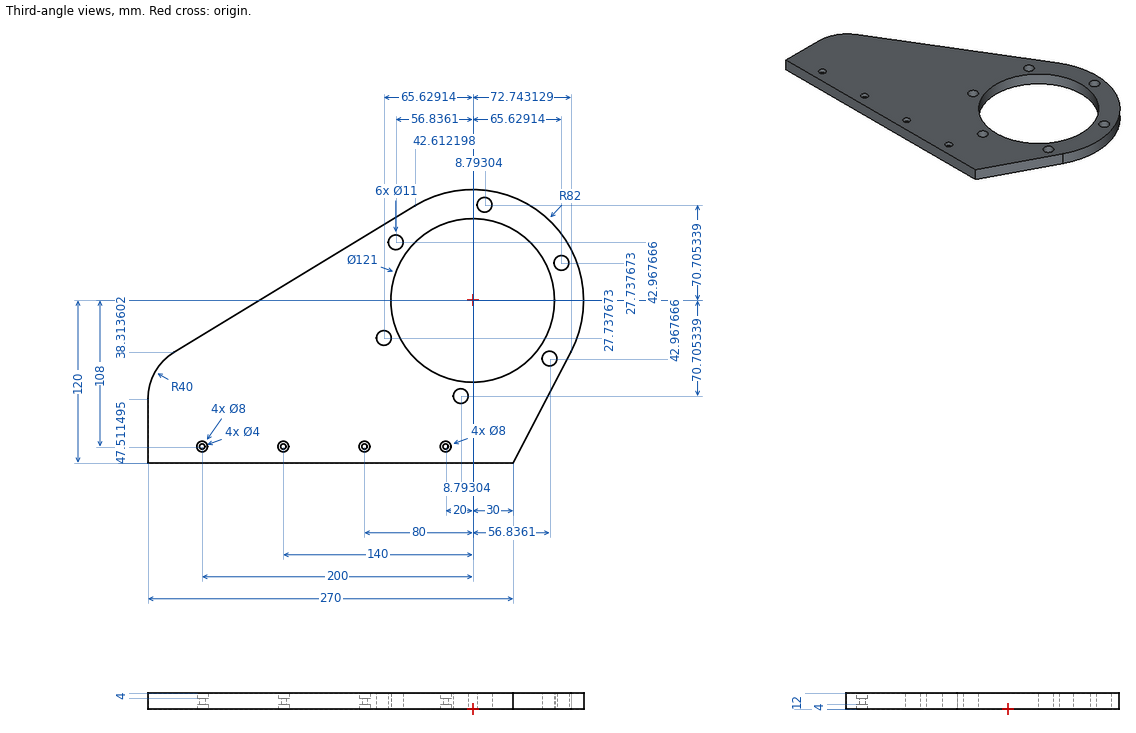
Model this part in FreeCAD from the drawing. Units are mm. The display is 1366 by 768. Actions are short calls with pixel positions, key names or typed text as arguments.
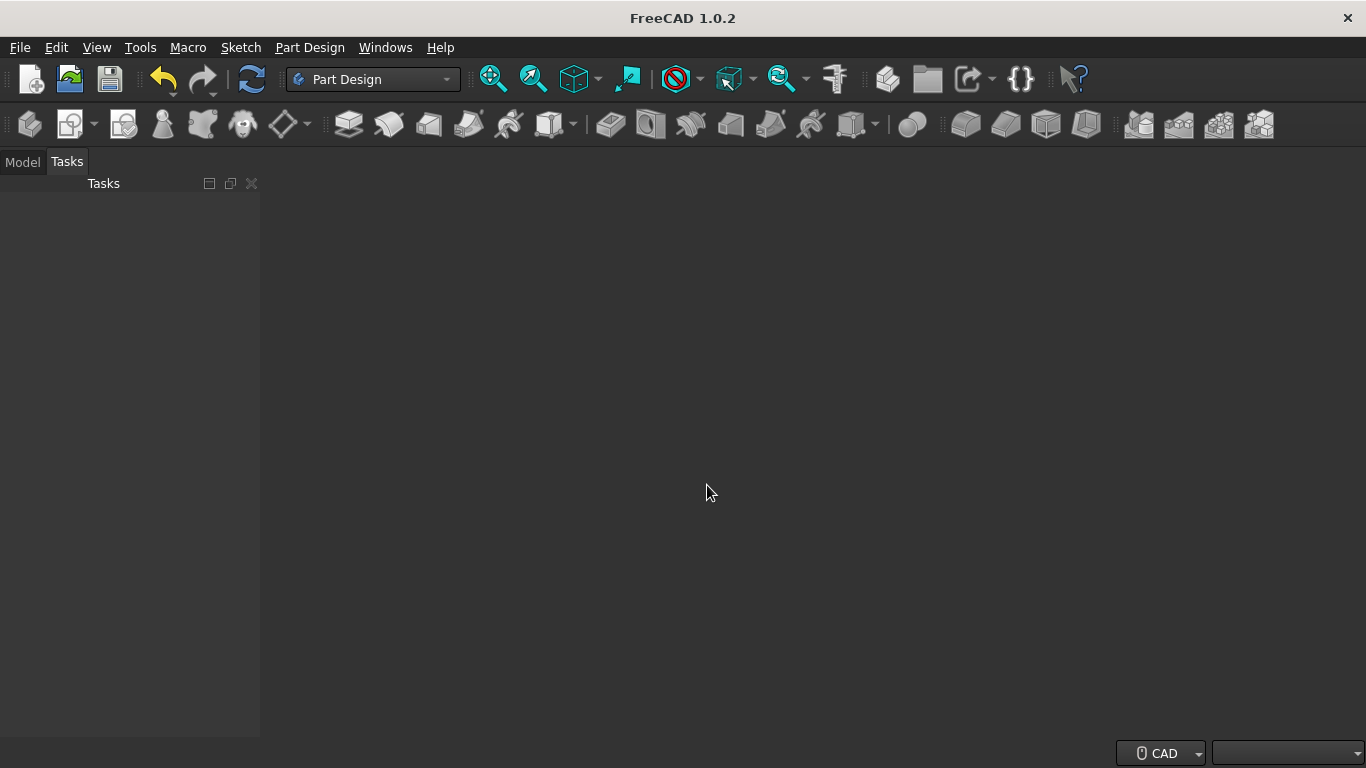
click(30, 80)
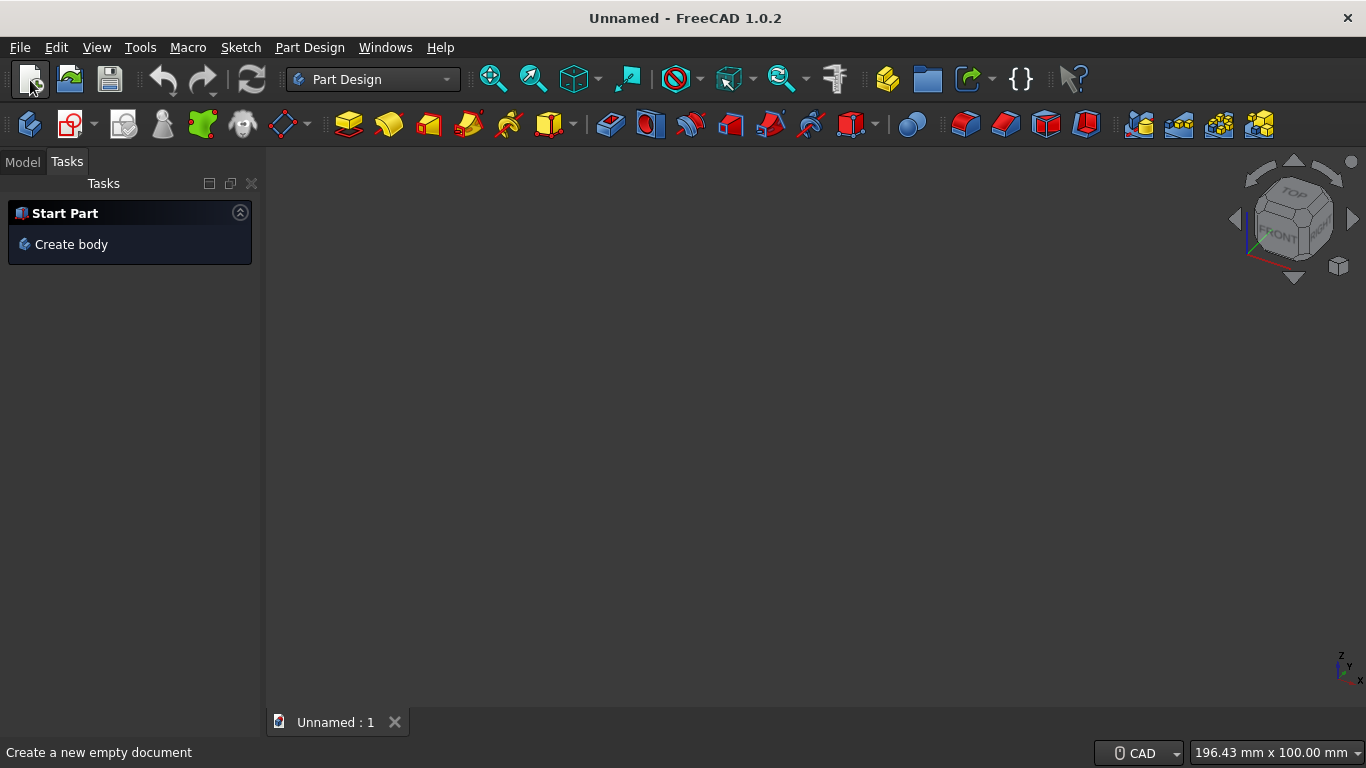
click(70, 124)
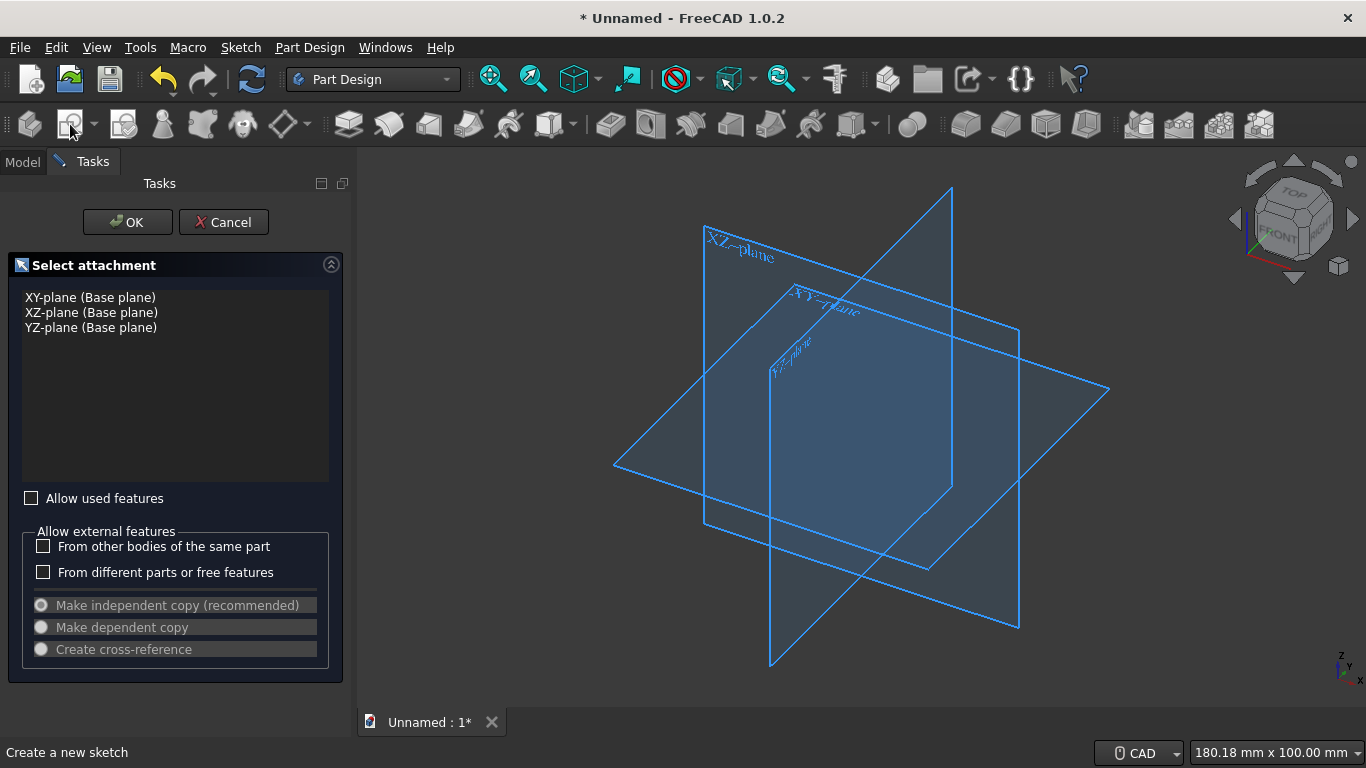
click(82, 298)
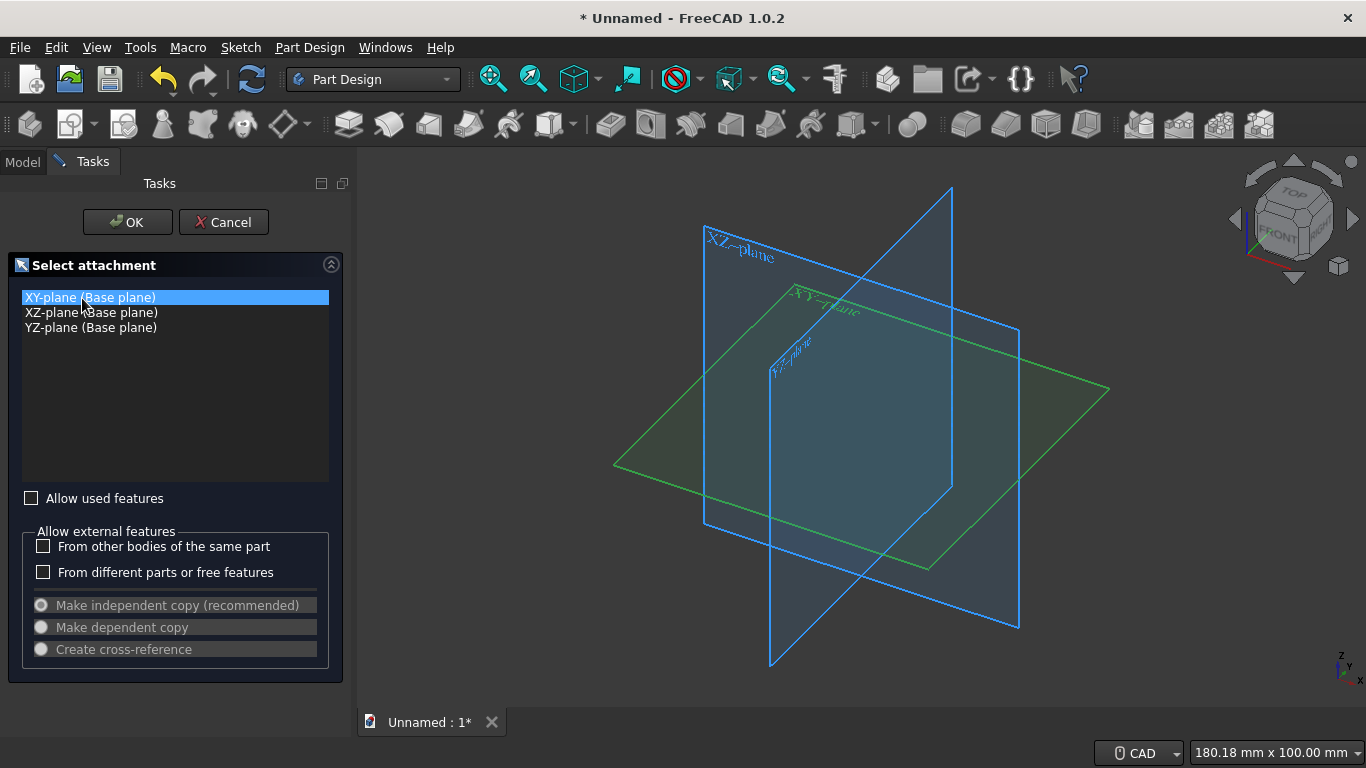
click(128, 222)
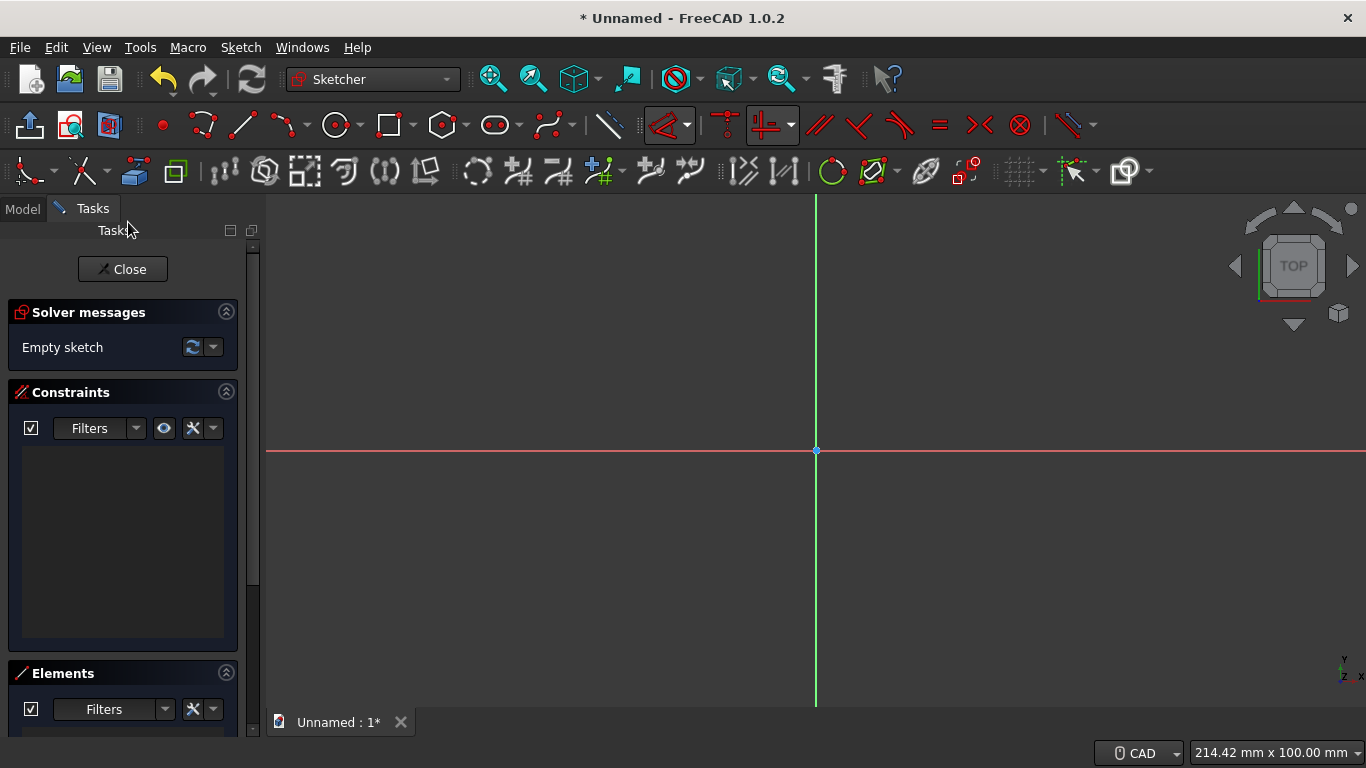
scroll(903, 395, down, 6)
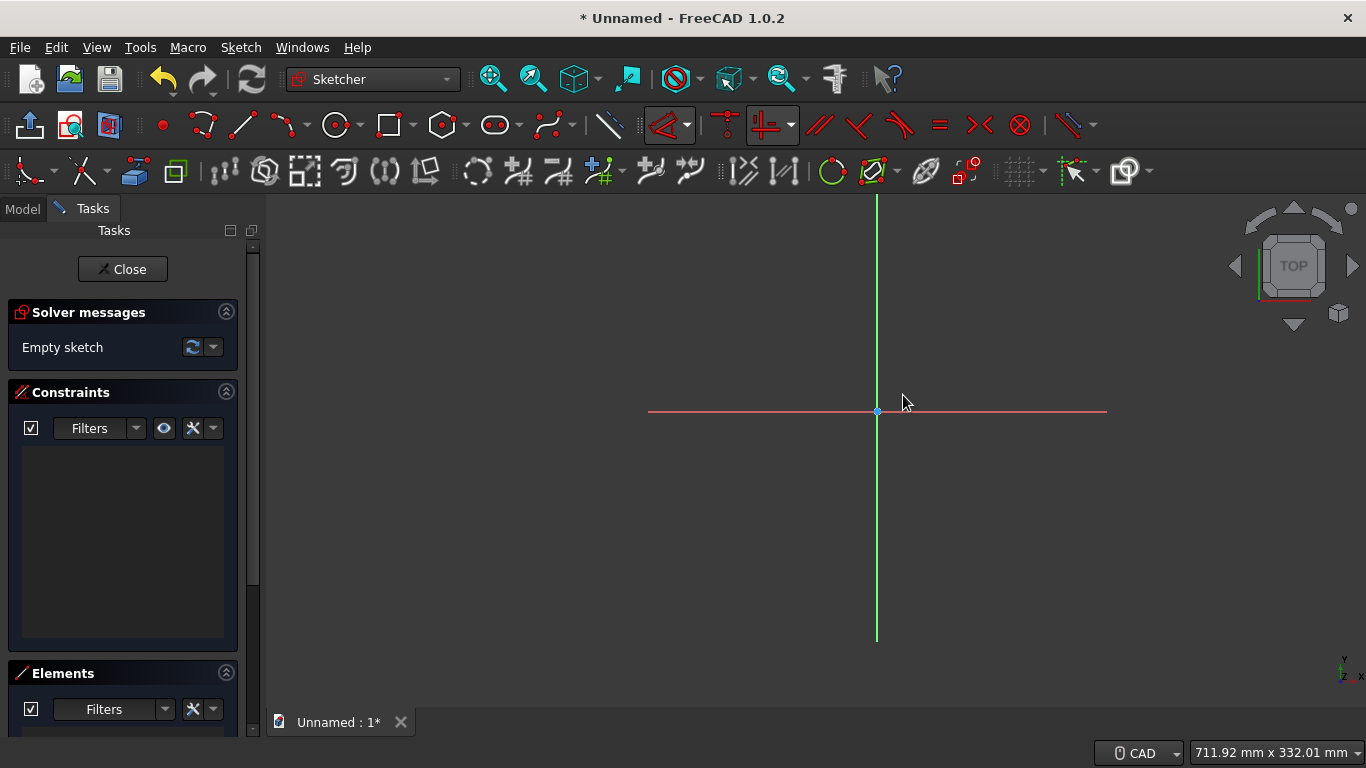
click(204, 126)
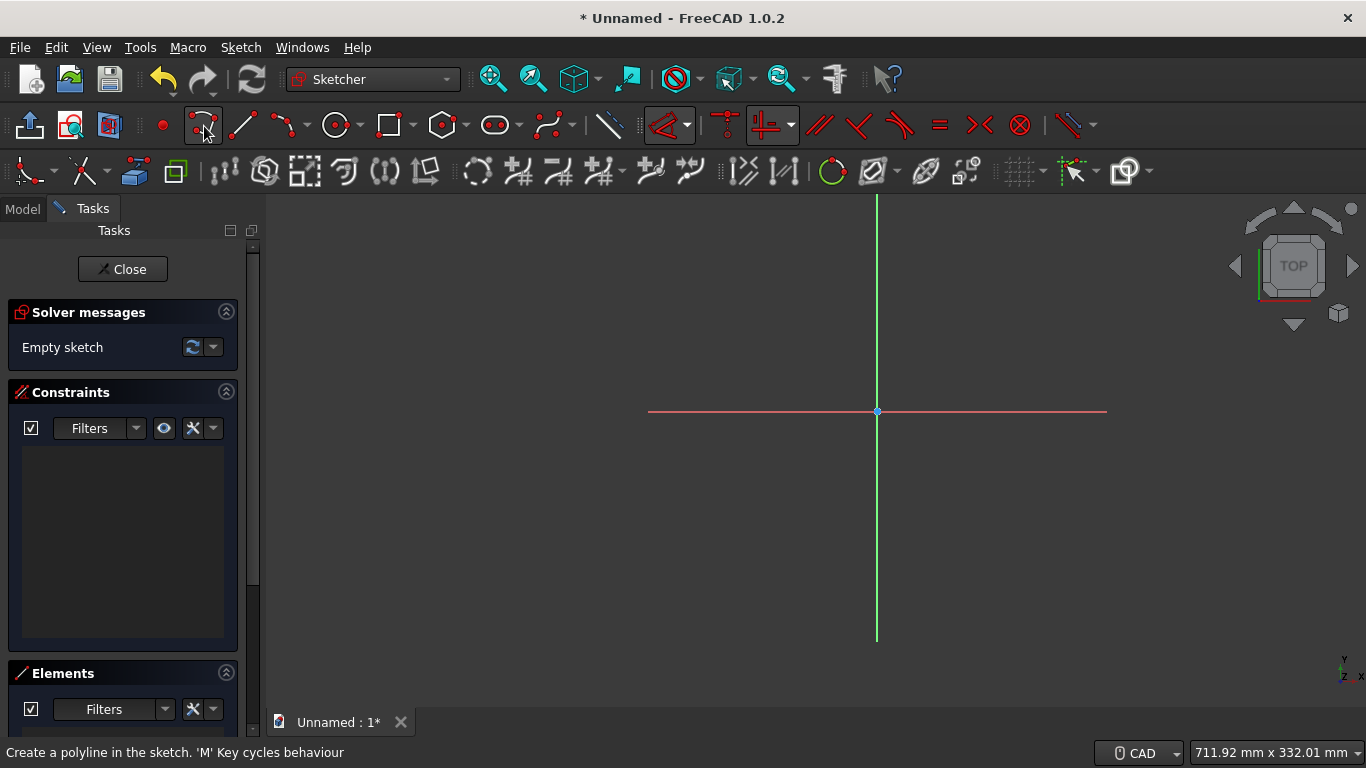
click(506, 524)
click(506, 597)
click(924, 597)
click(990, 470)
right_click(990, 470)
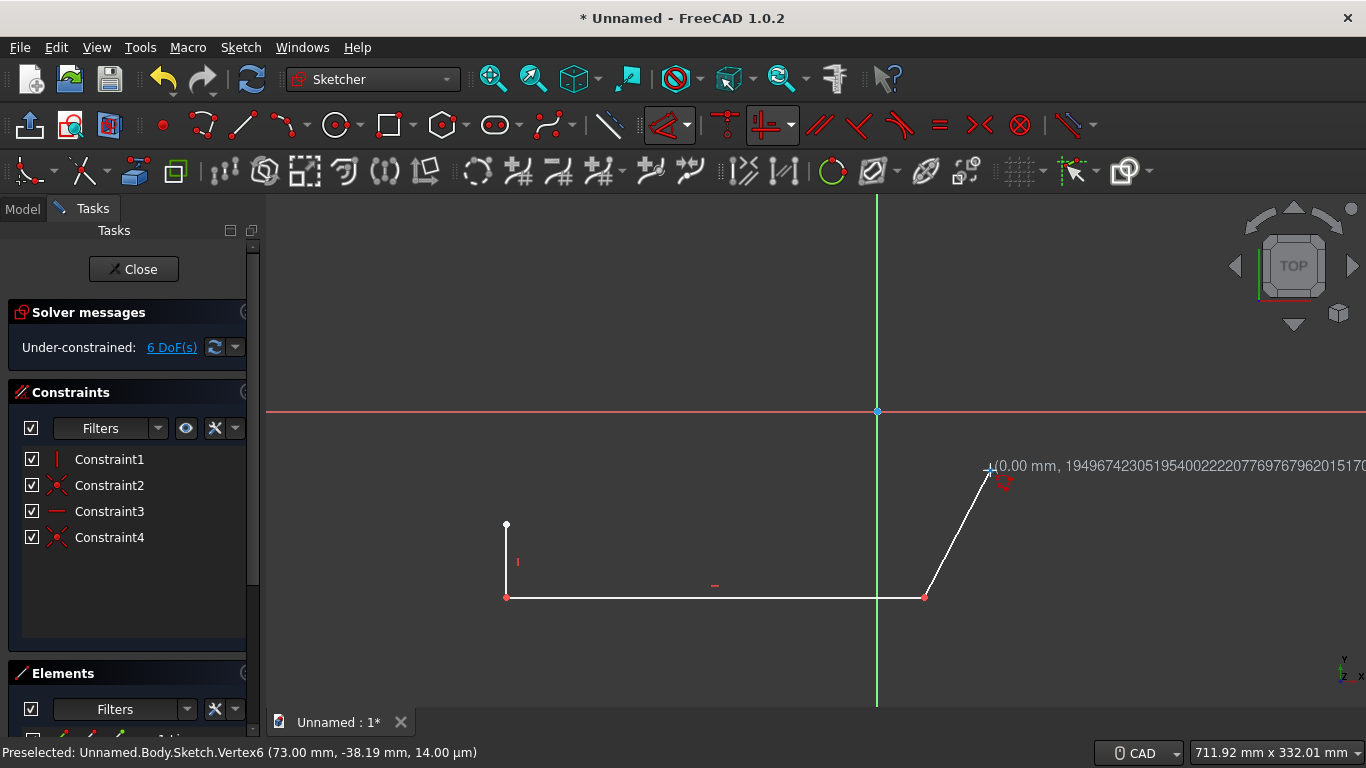
click(244, 126)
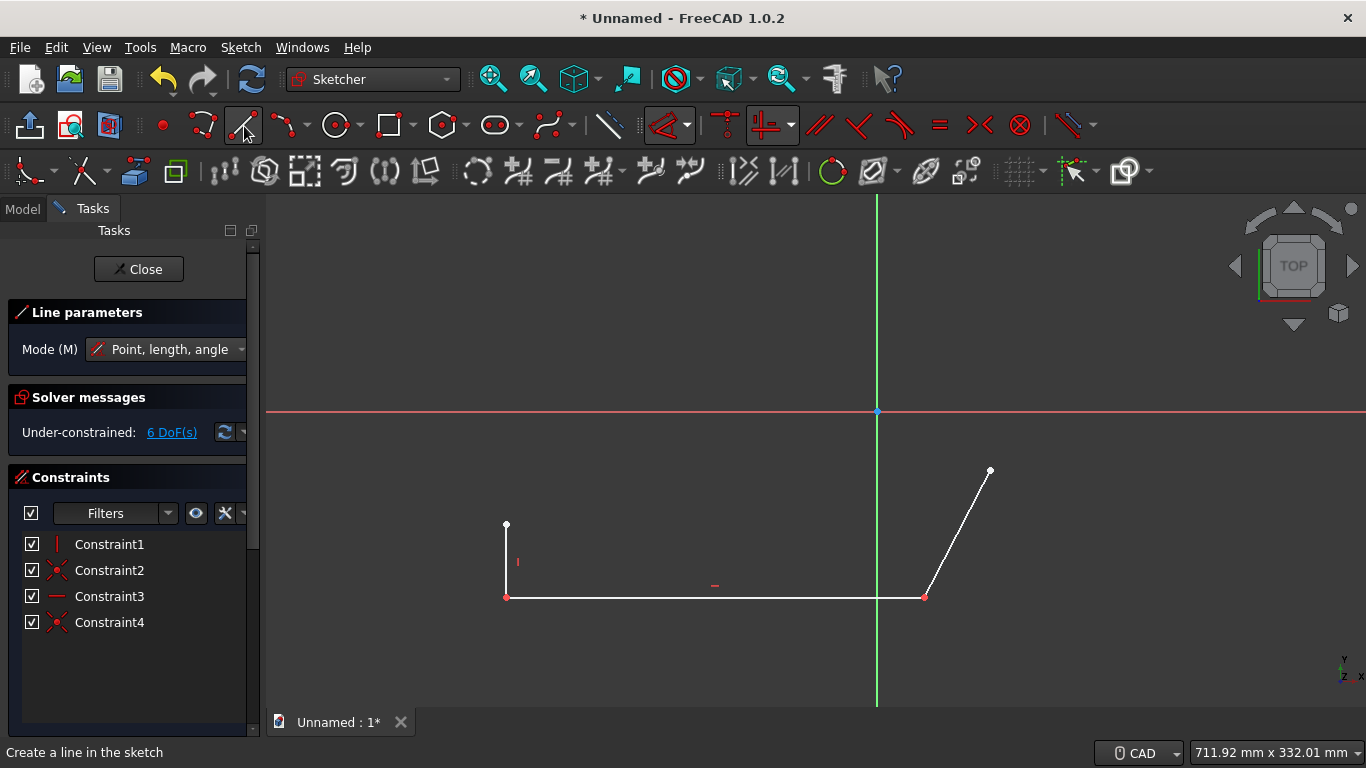
click(811, 304)
click(536, 471)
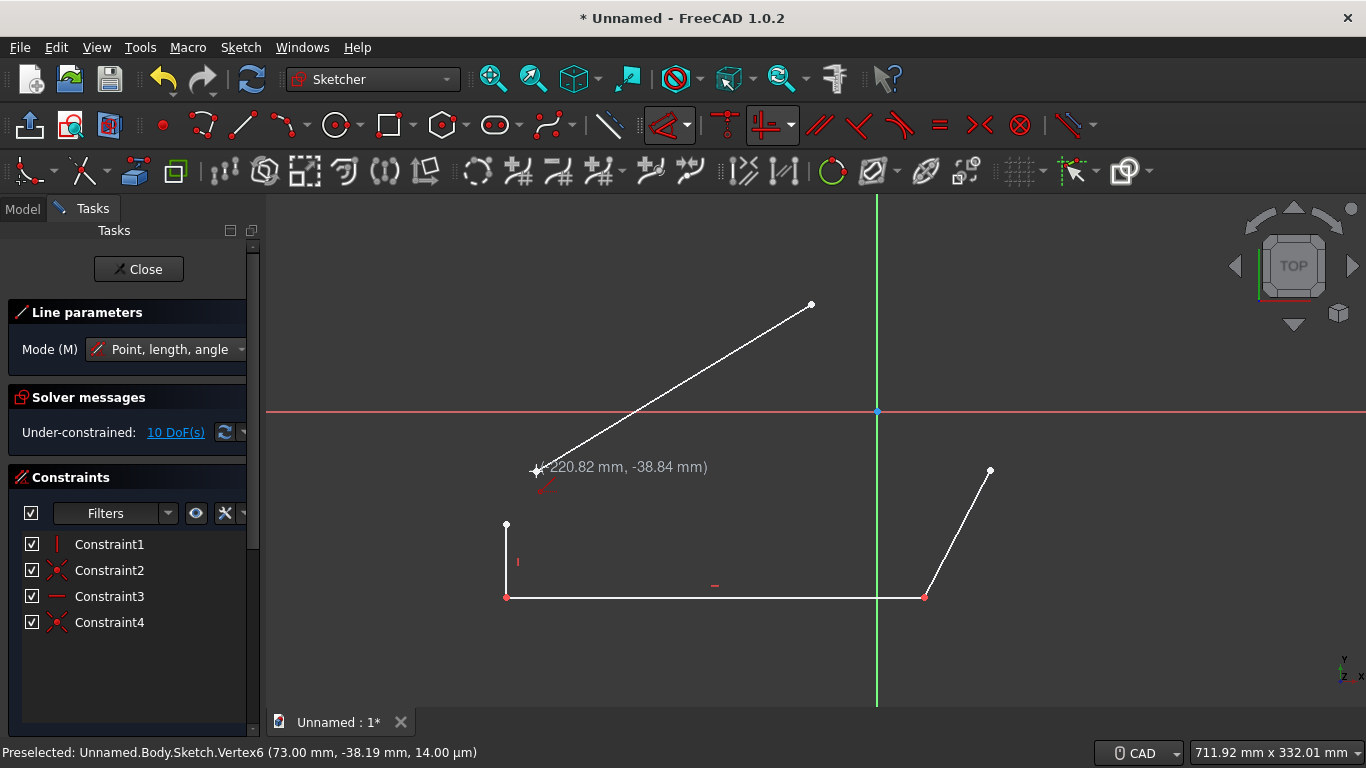
click(284, 126)